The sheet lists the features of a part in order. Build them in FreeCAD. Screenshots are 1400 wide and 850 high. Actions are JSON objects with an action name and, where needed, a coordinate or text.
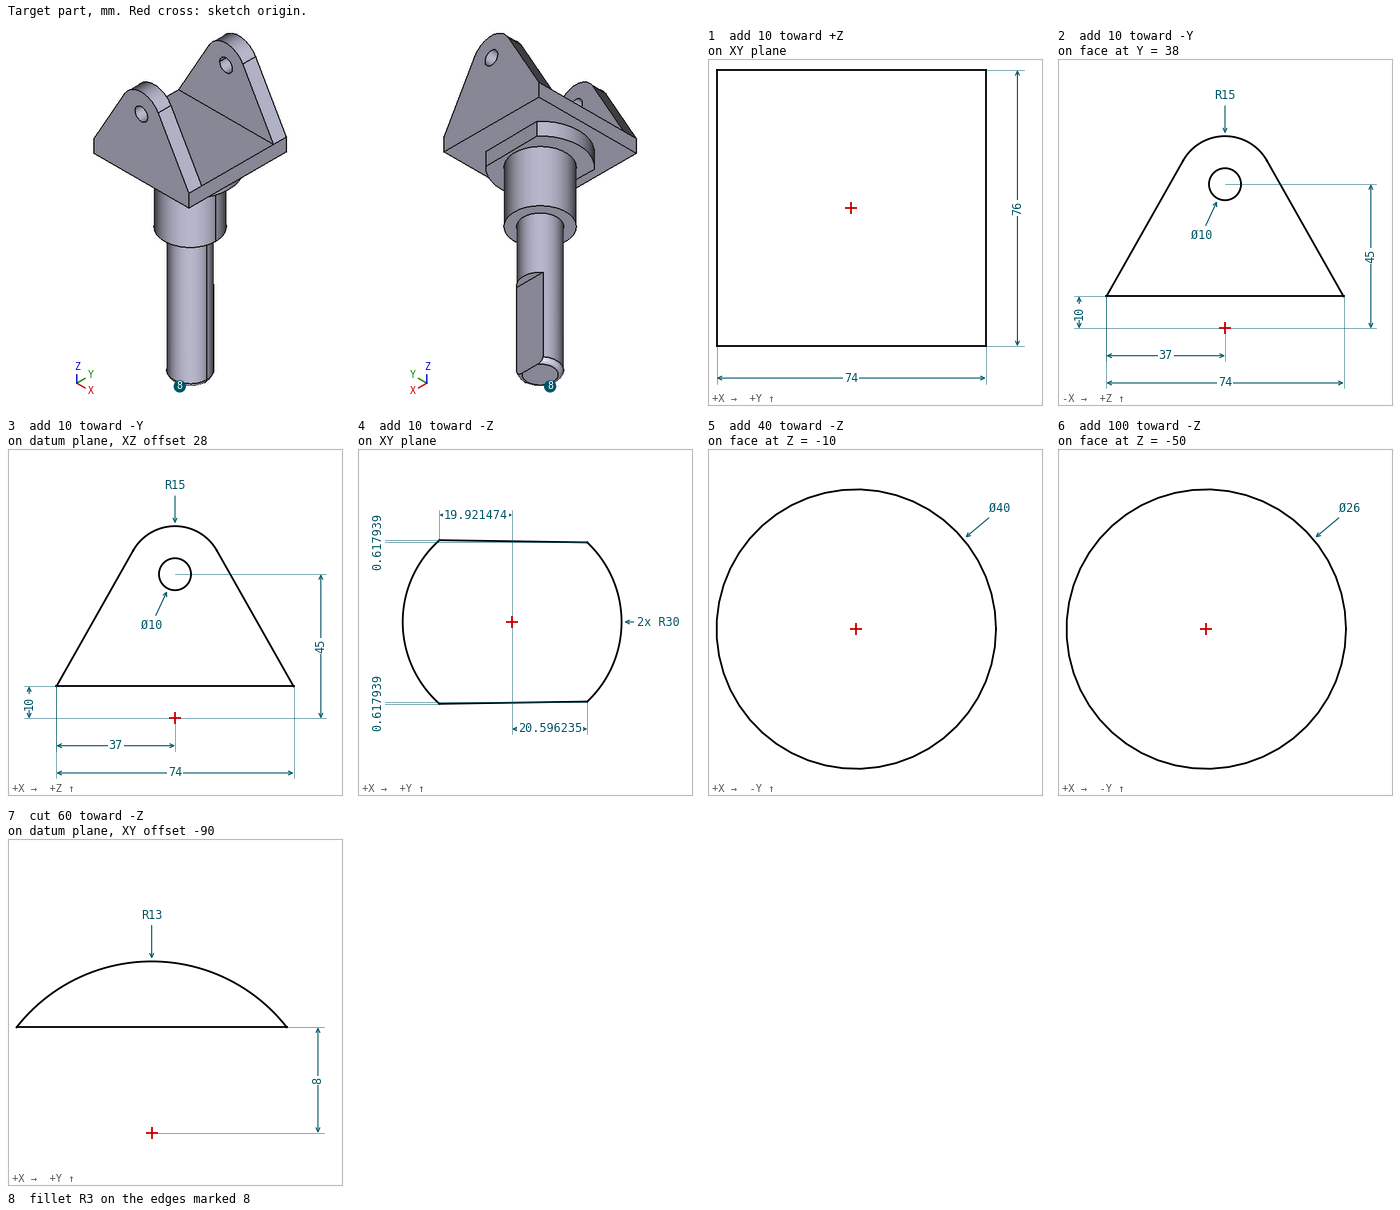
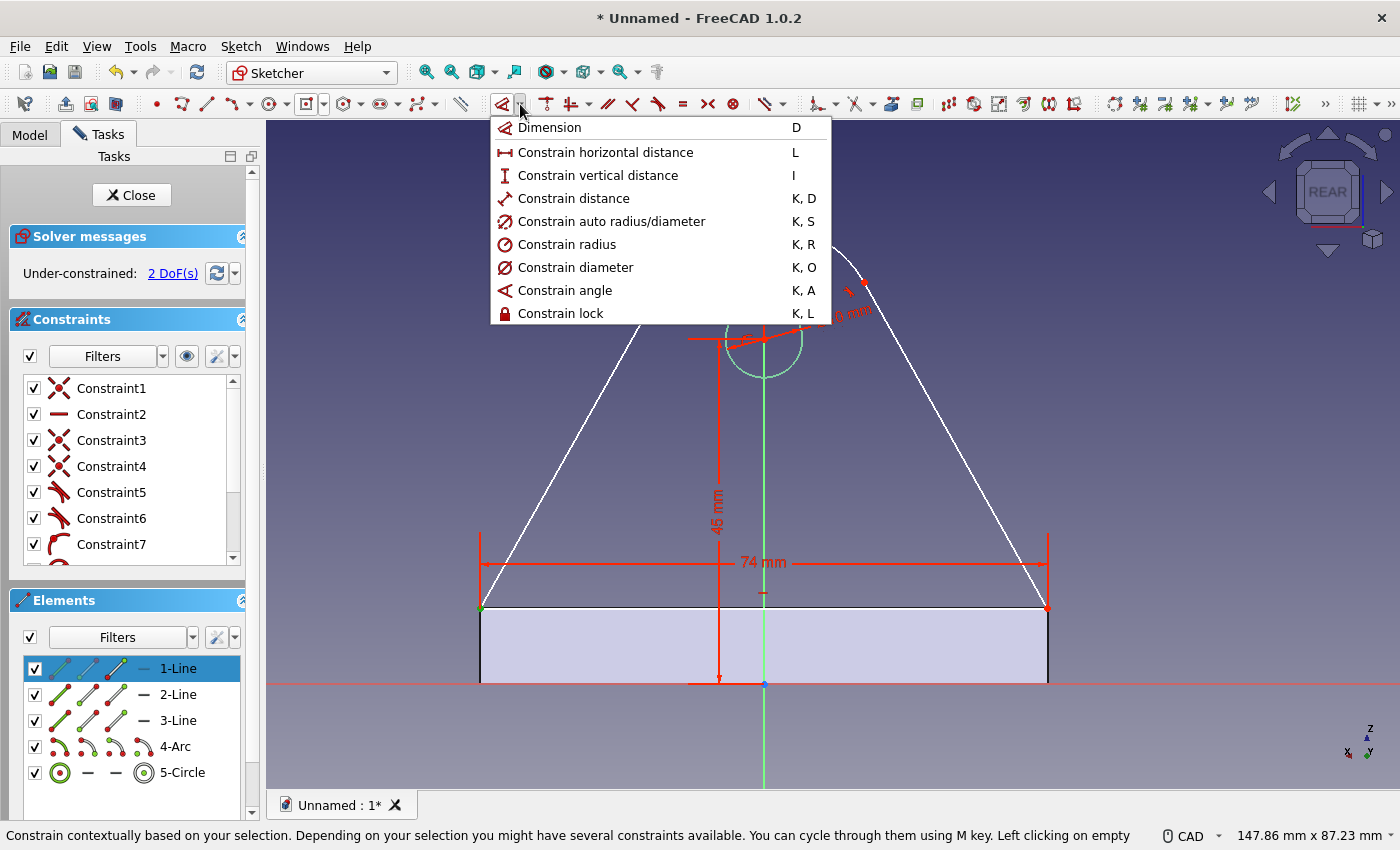
{"action": "left_click", "coordinate": [661, 152]}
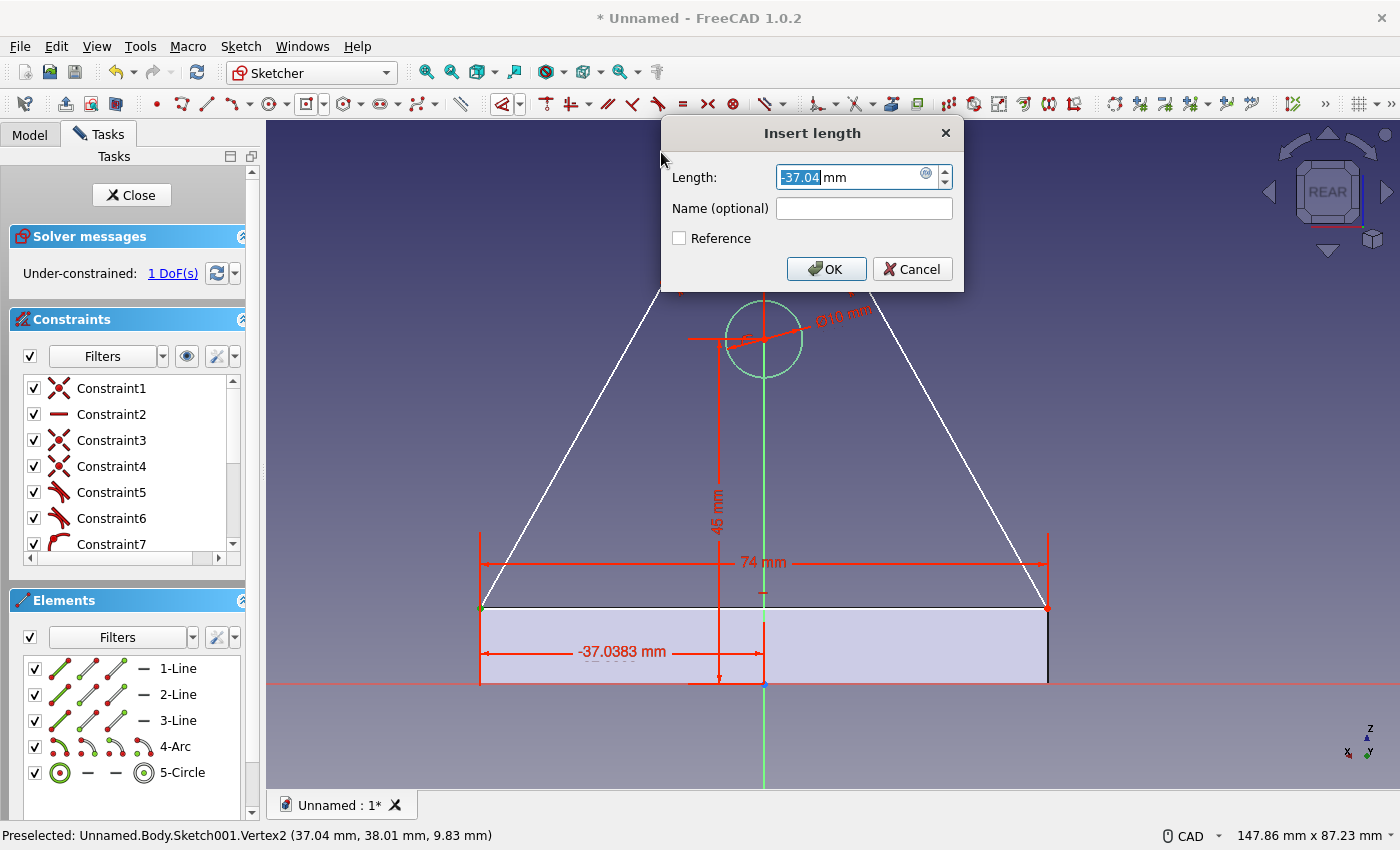
{"action": "type", "text": "-37"}
{"action": "key", "text": "Return"}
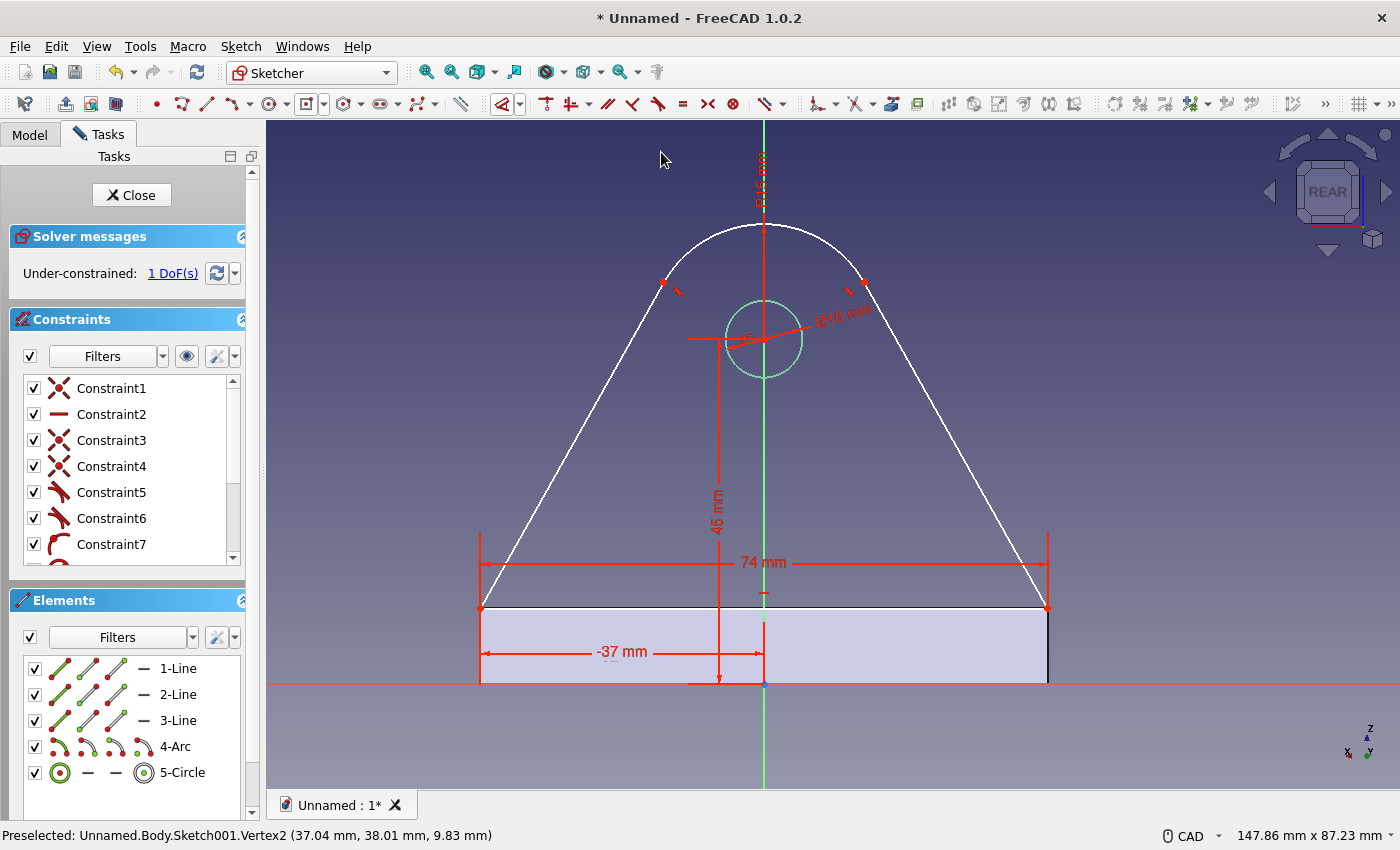
{"action": "left_click", "coordinate": [480, 609]}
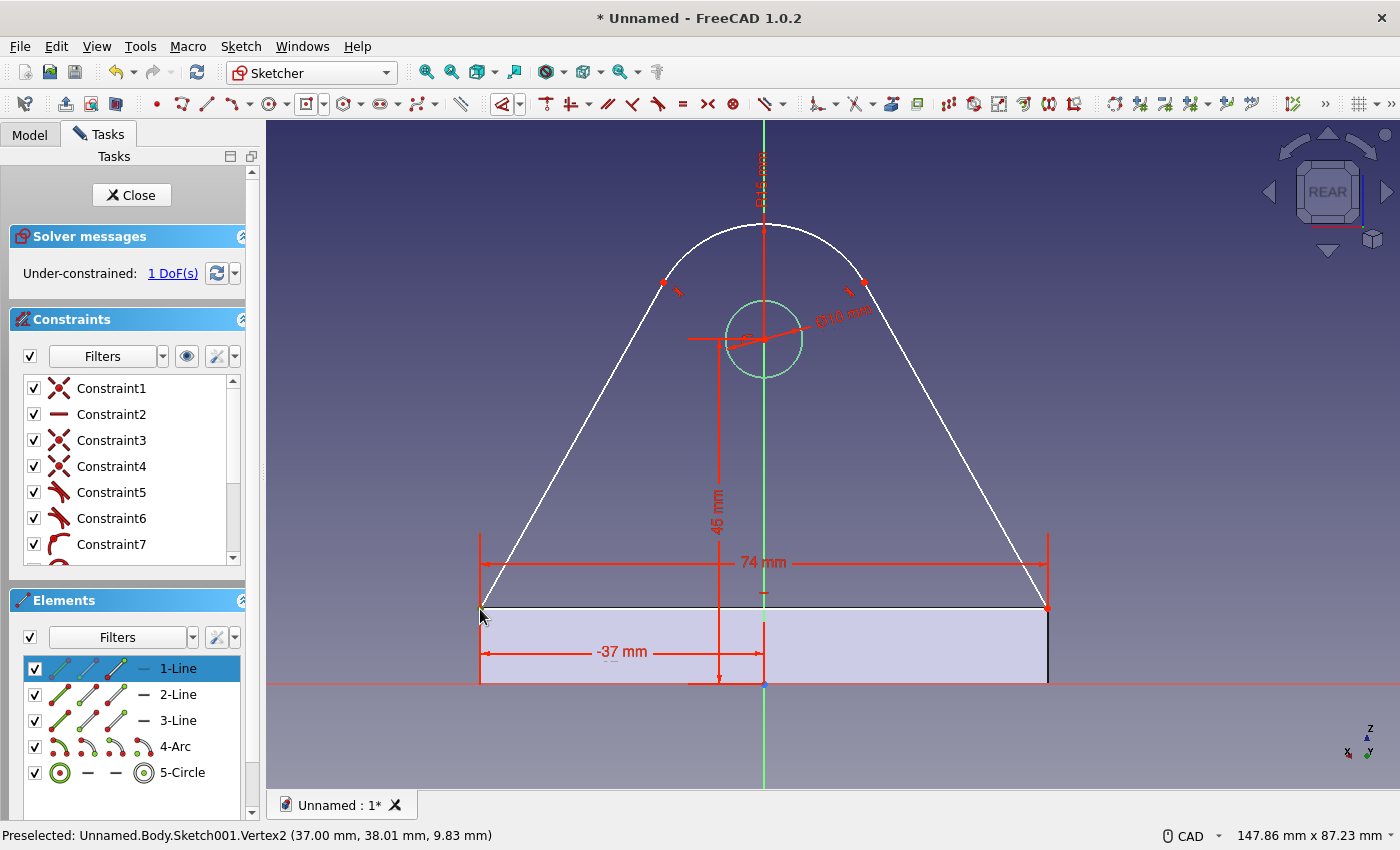
{"action": "key", "text": "i"}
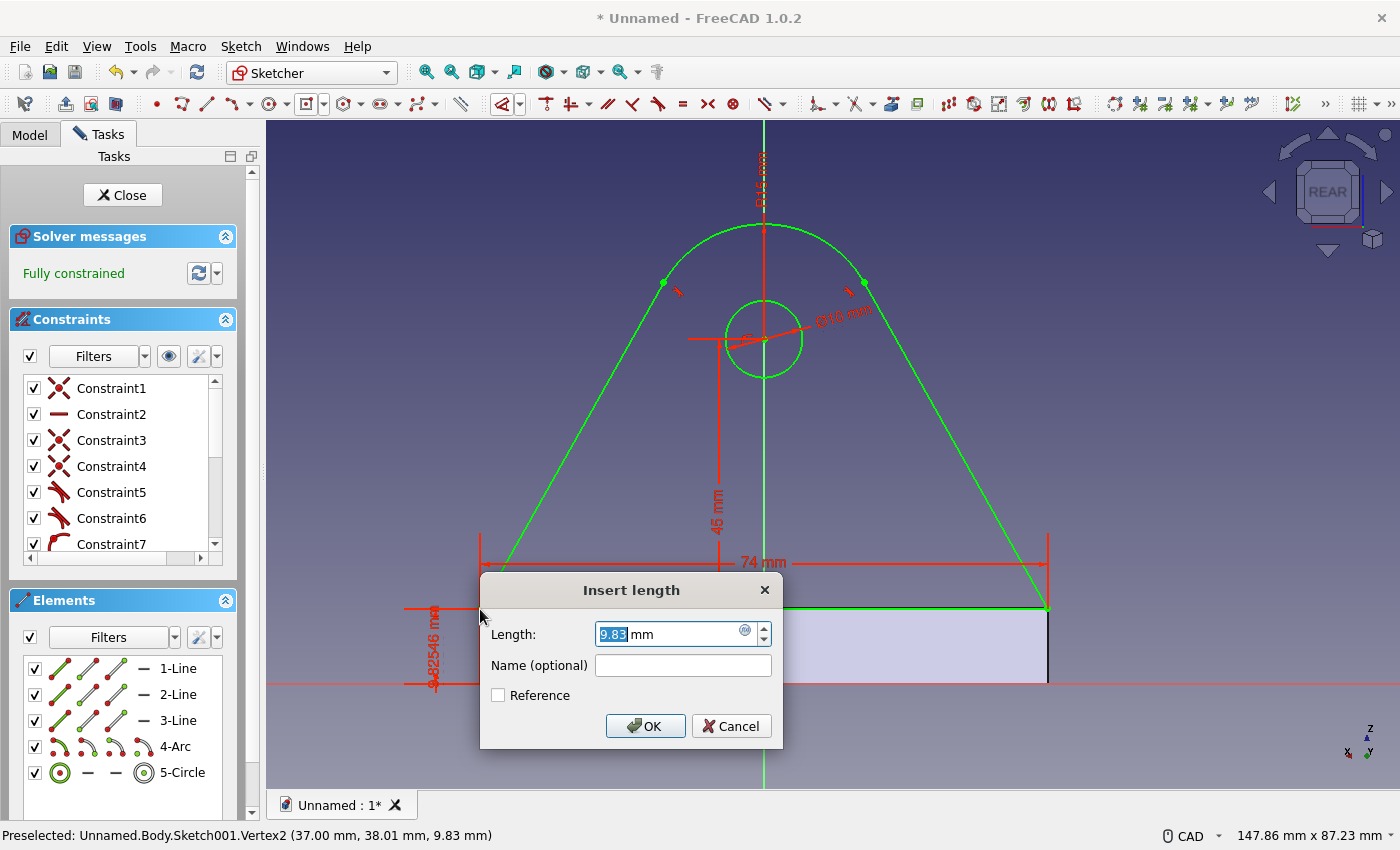
{"action": "type", "text": "10"}
{"action": "key", "text": "Return"}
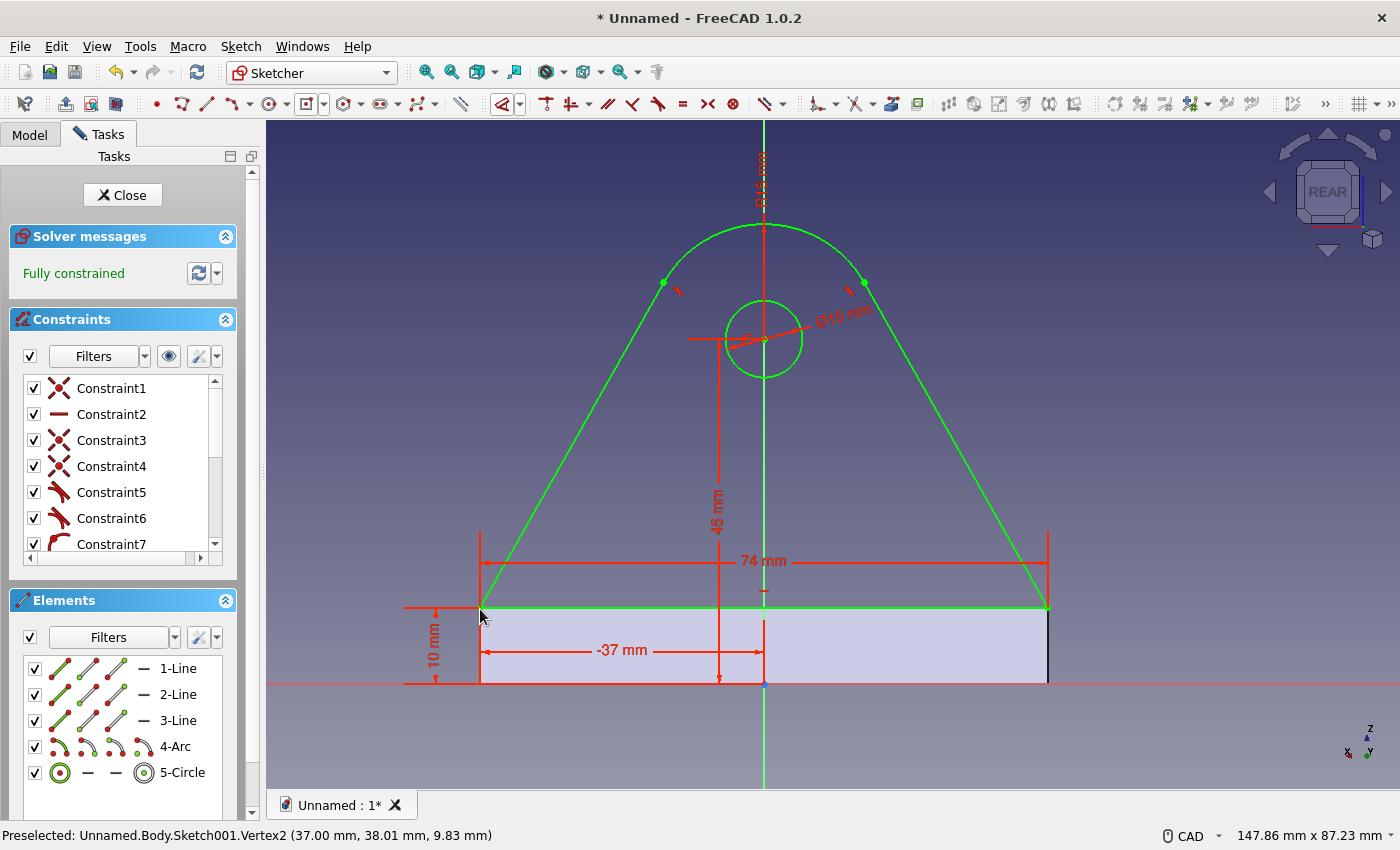
{"action": "left_click", "coordinate": [123, 195]}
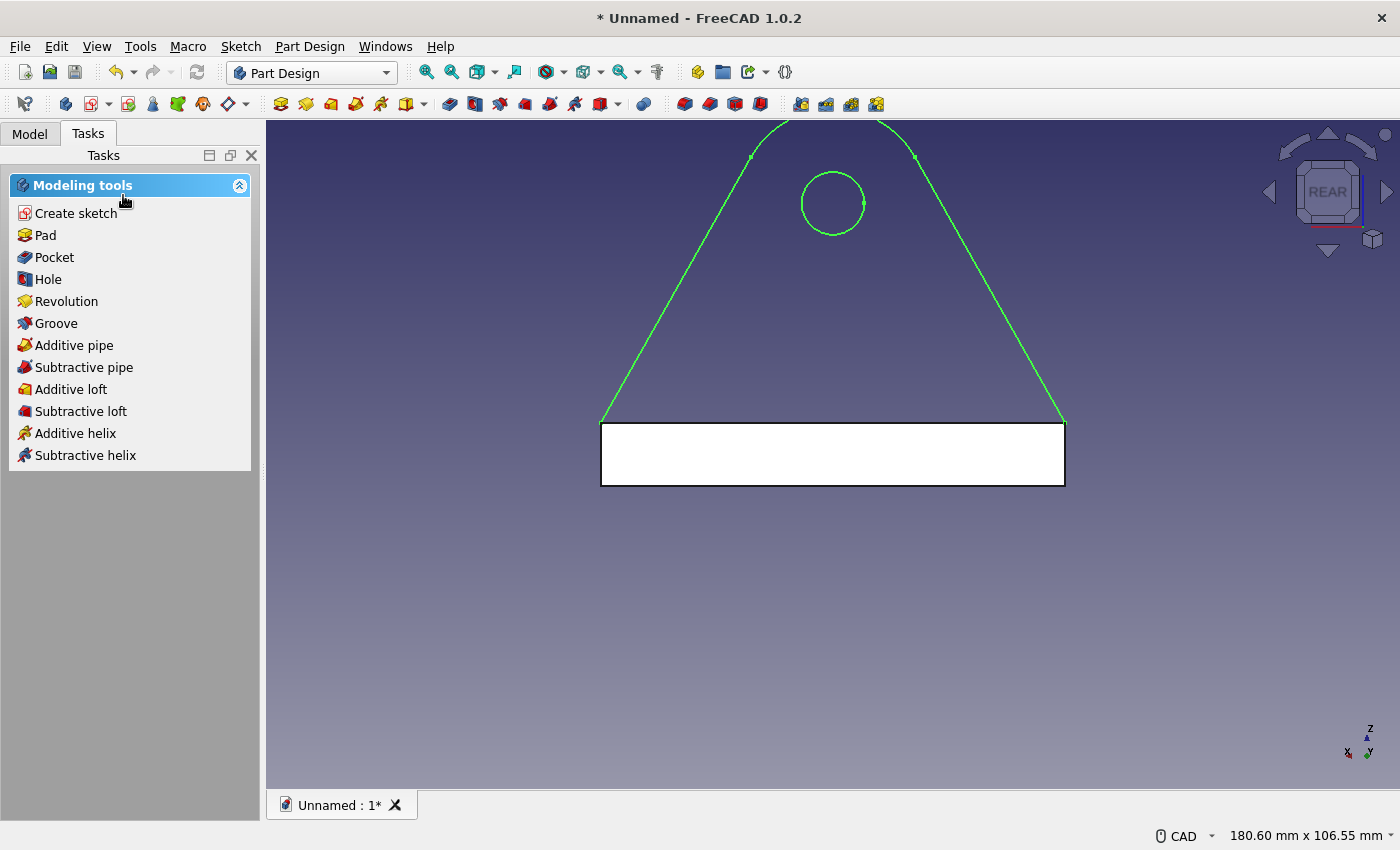
{"action": "left_click", "coordinate": [281, 104]}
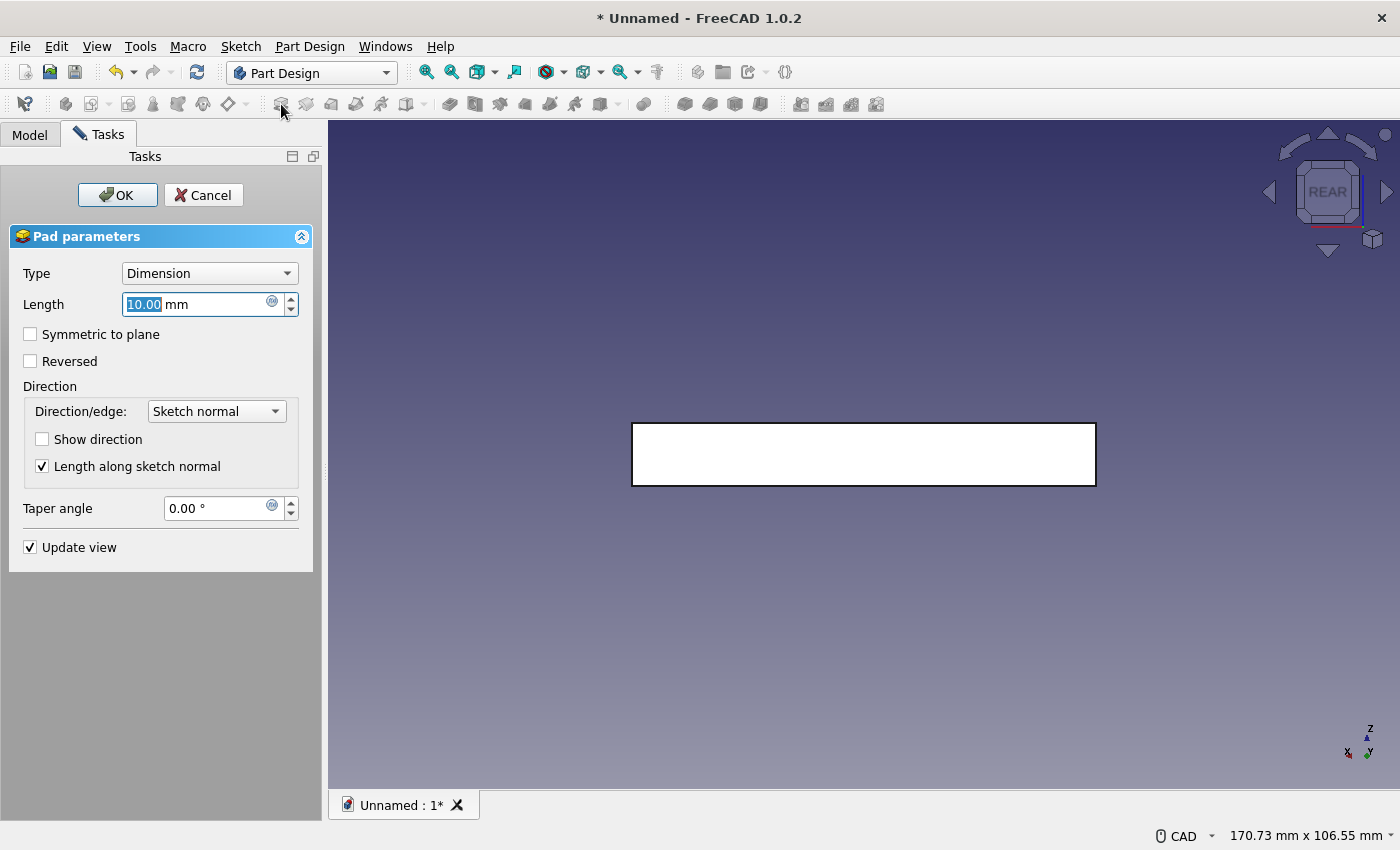
{"action": "type", "text": "10"}
{"action": "key", "text": "Tab"}